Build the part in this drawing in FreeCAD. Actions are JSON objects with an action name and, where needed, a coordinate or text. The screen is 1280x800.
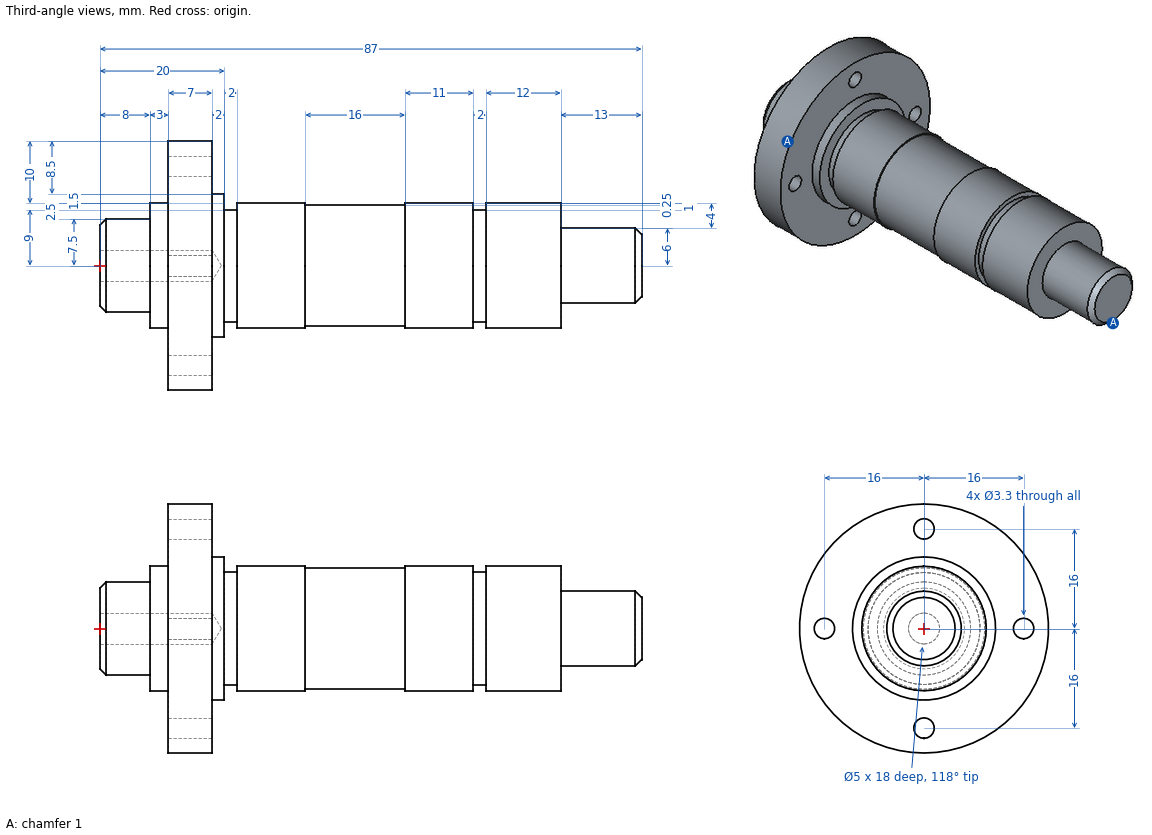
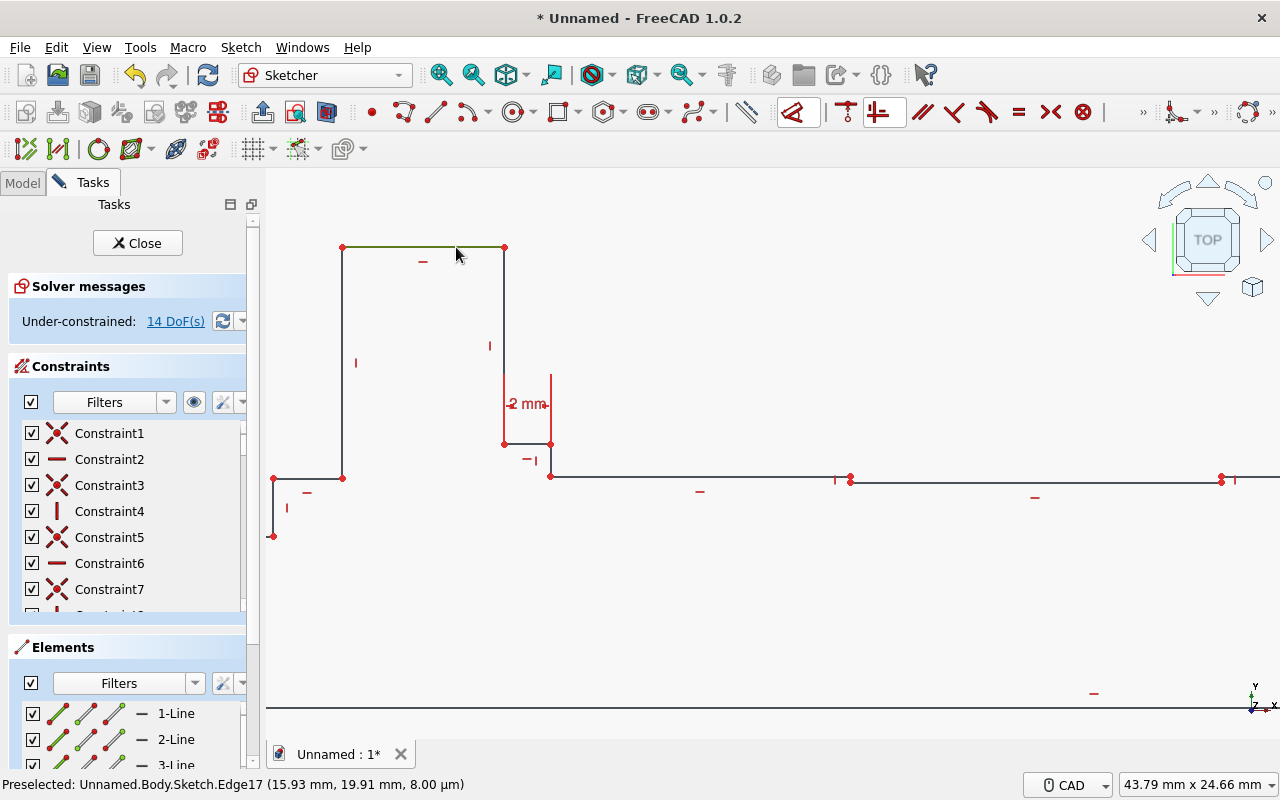
{"action": "left_click", "coordinate": [814, 112]}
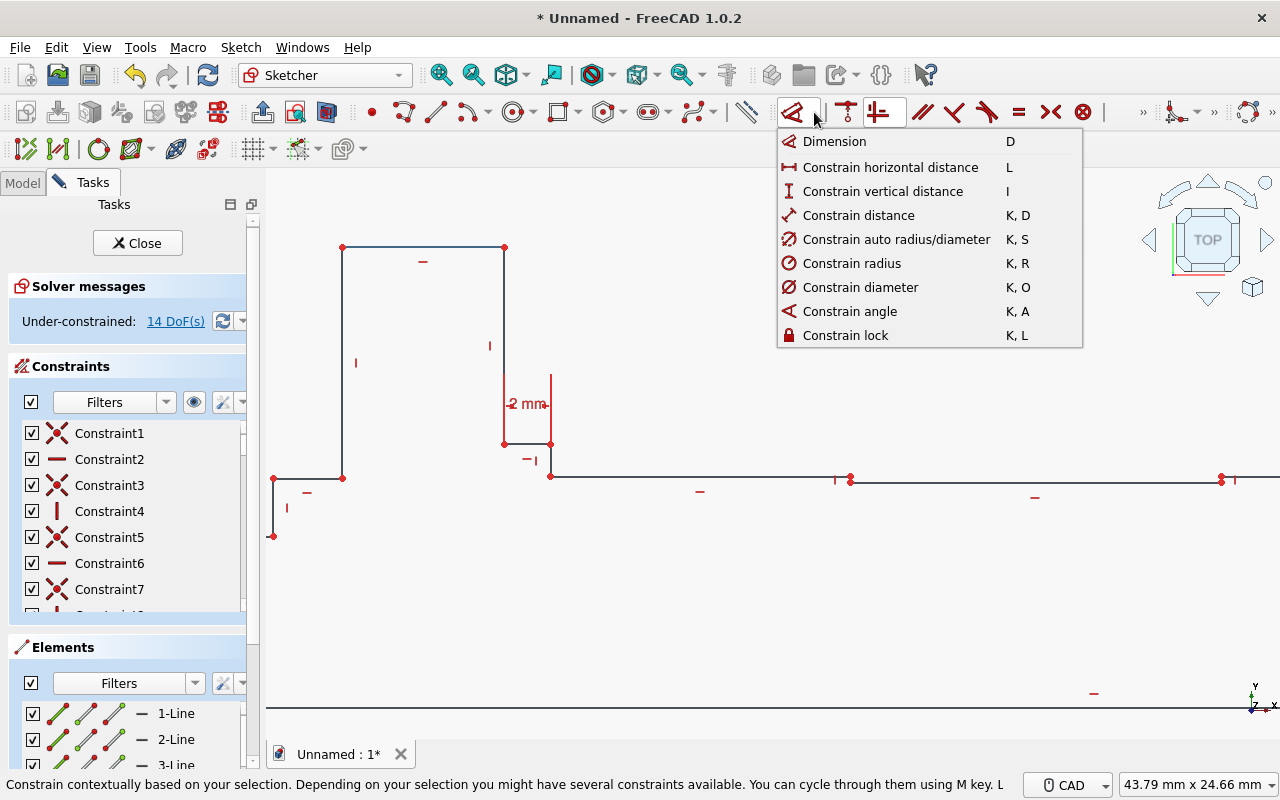
{"action": "left_click", "coordinate": [930, 167]}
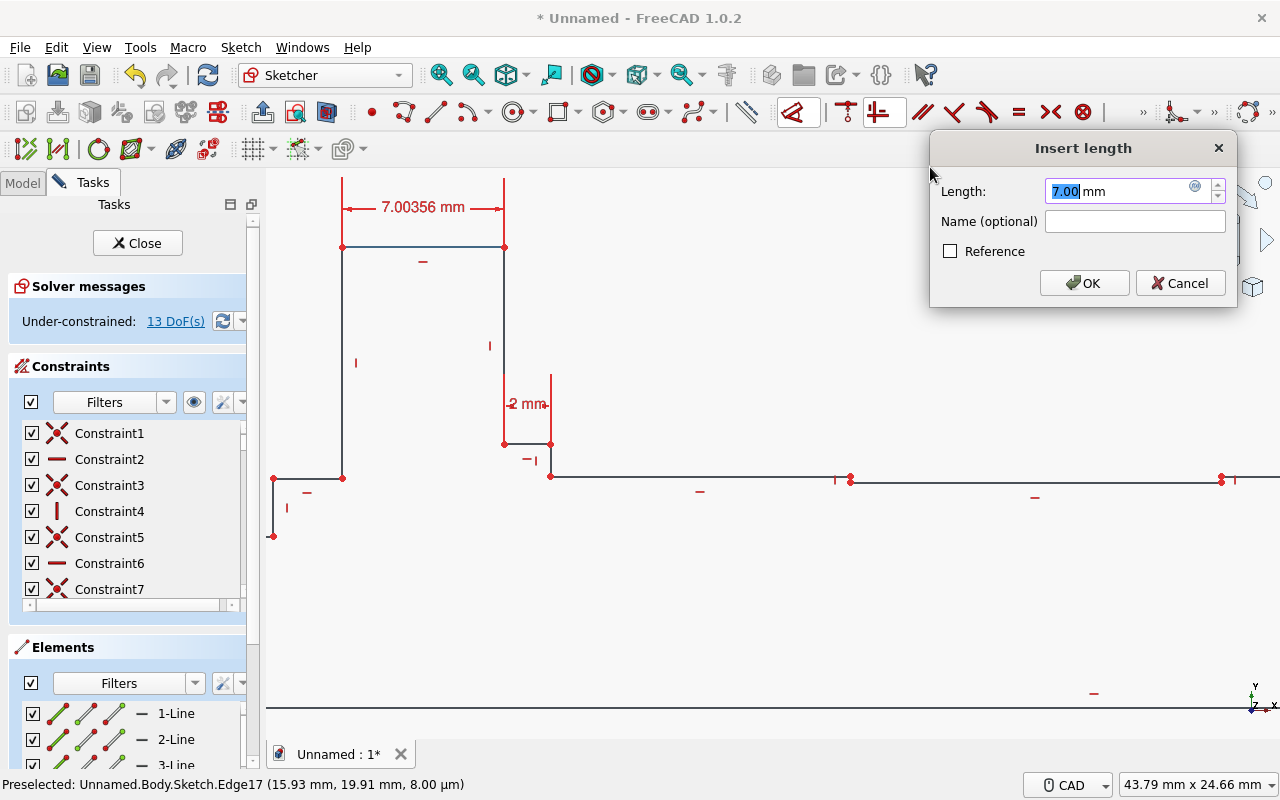
{"action": "type", "text": "7"}
{"action": "key", "text": "Return"}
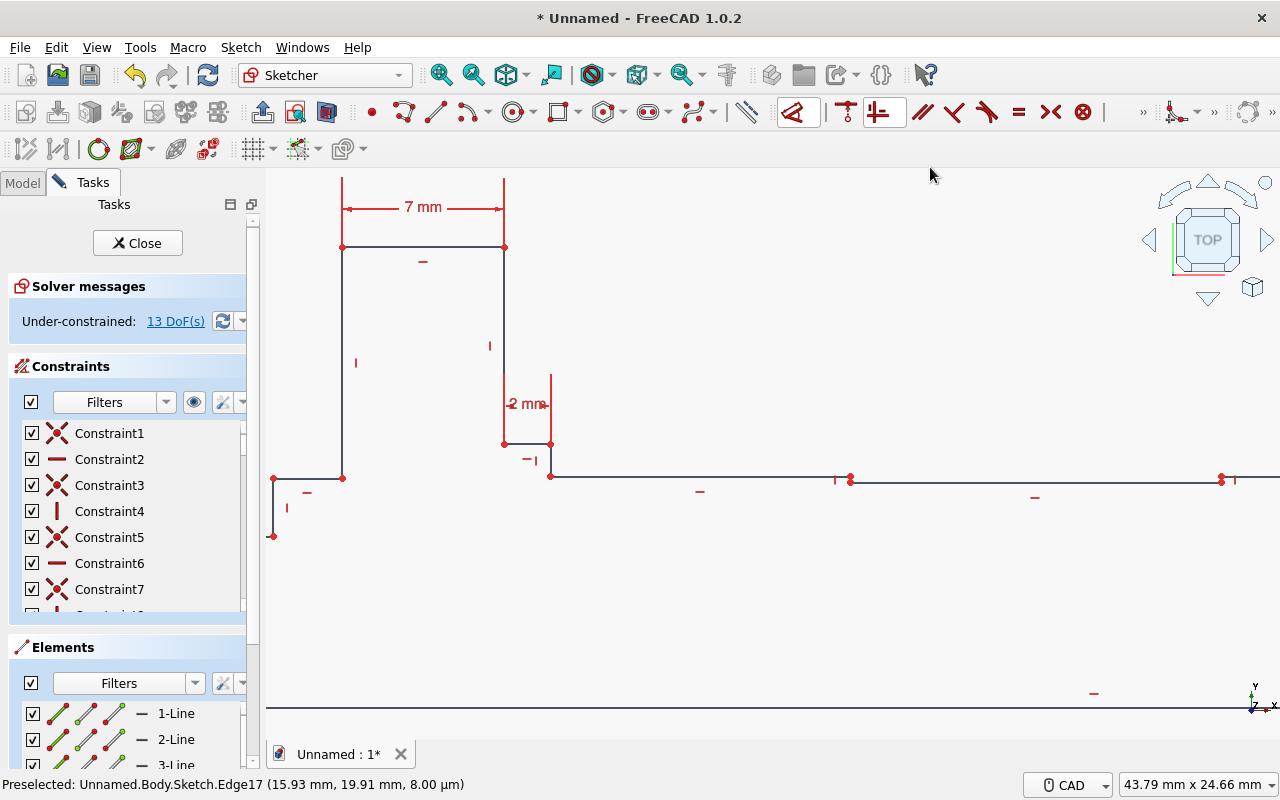
{"action": "left_click", "coordinate": [321, 479]}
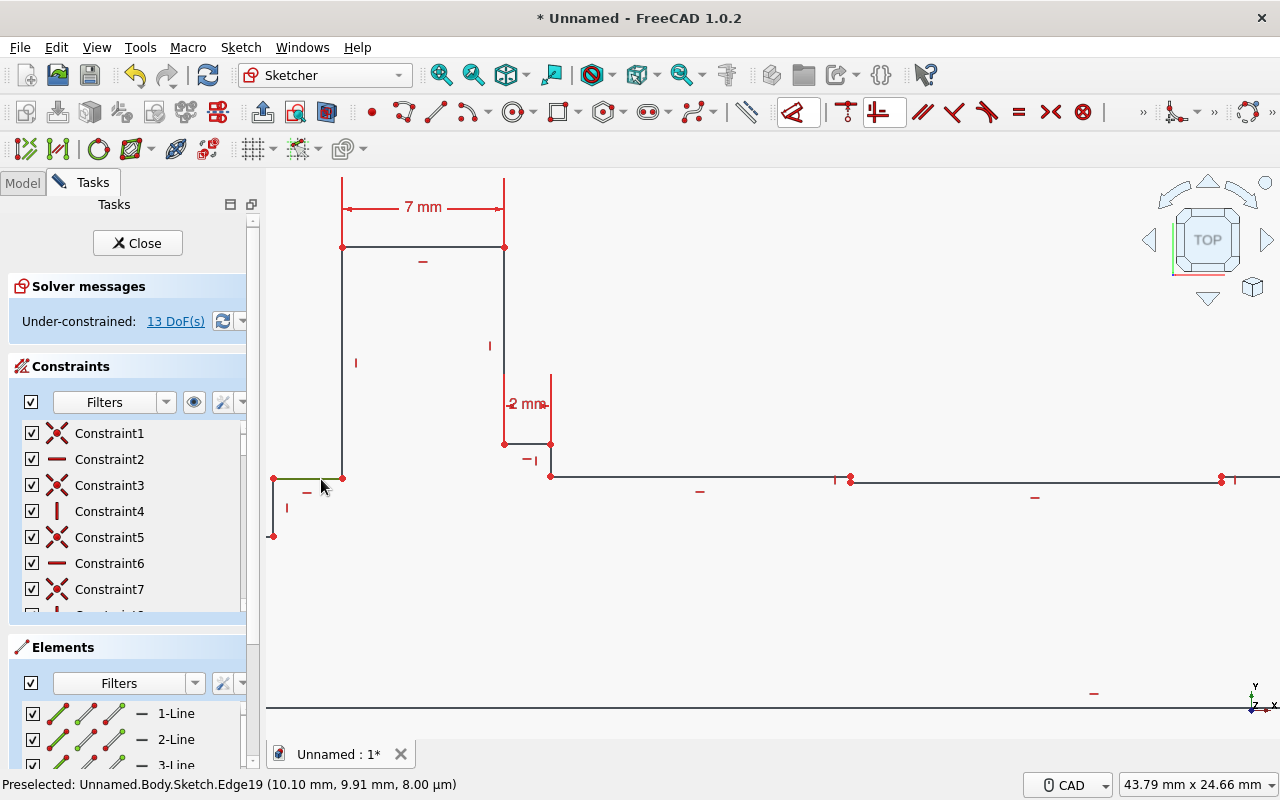
{"action": "key", "text": "l"}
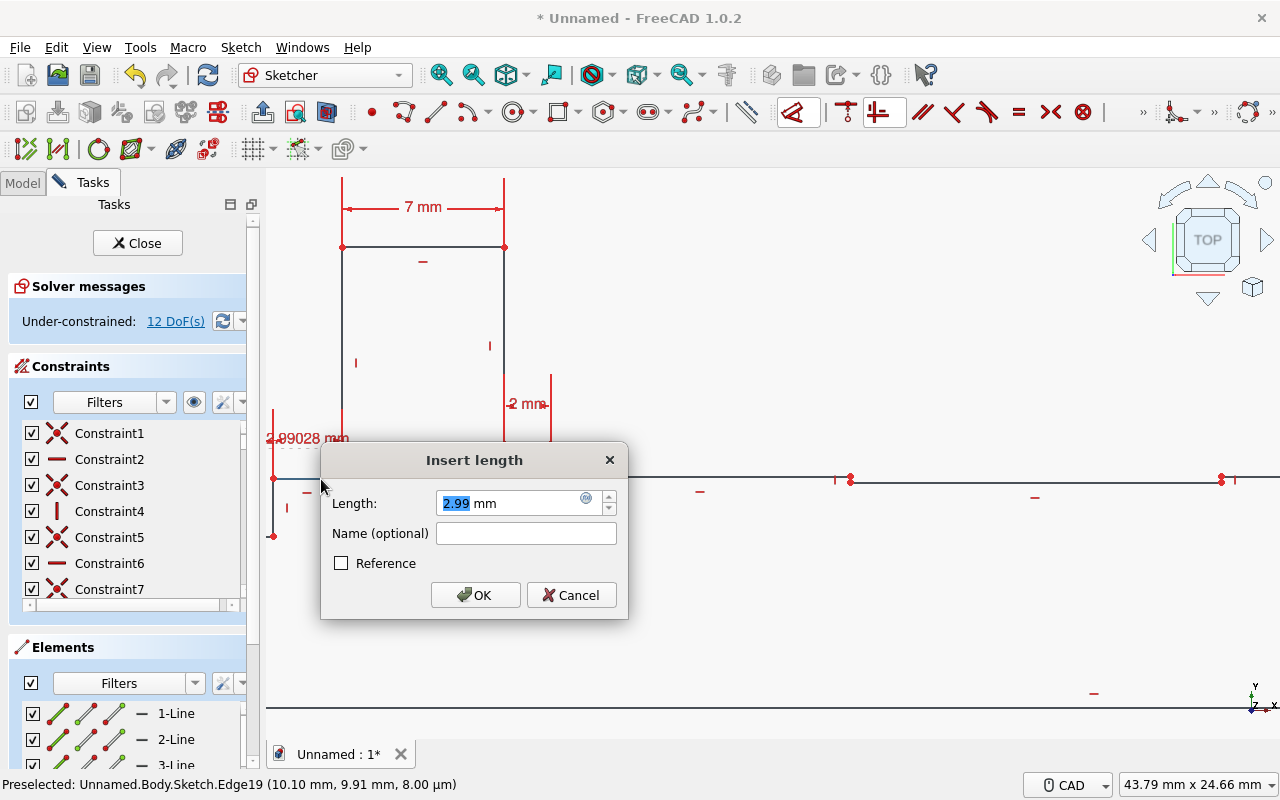
{"action": "type", "text": "3"}
{"action": "key", "text": "Return"}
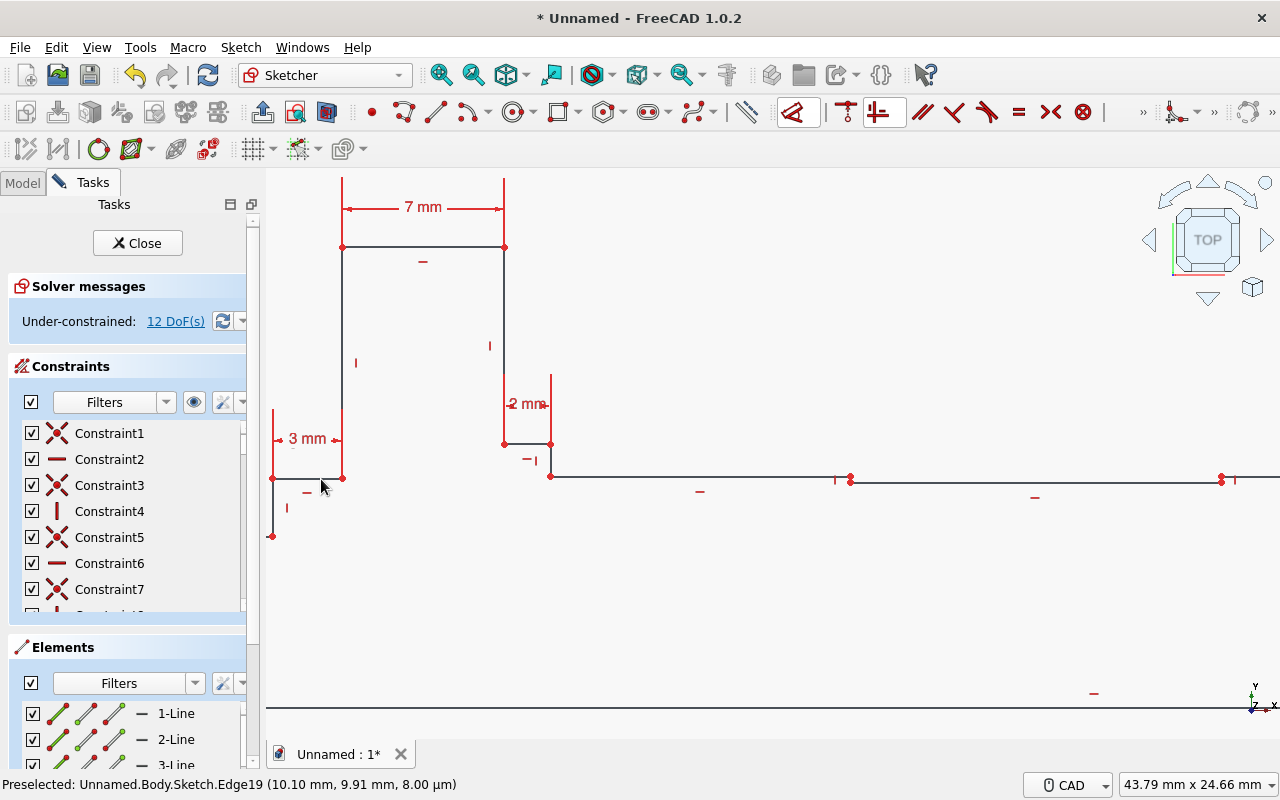
{"action": "scroll", "coordinate": [536, 444], "scroll_direction": "down", "scroll_amount": 6}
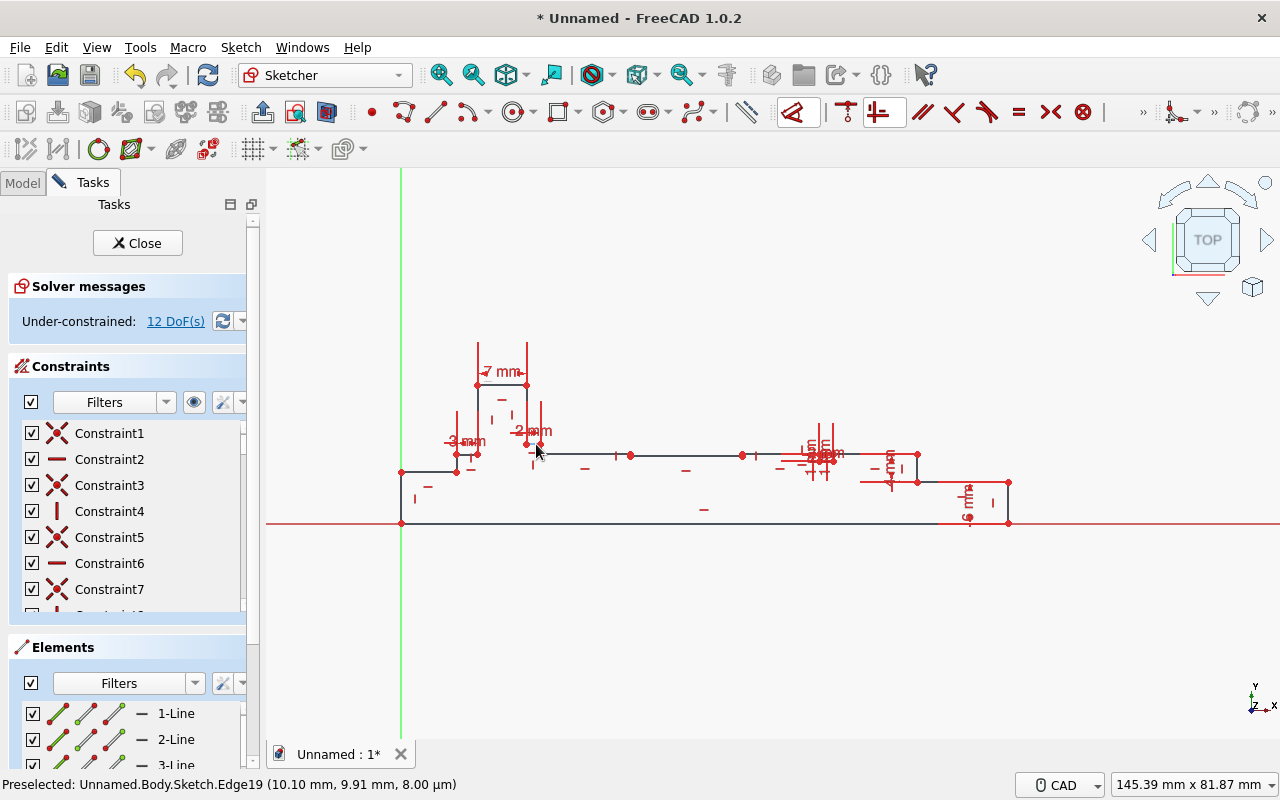
{"action": "left_click", "coordinate": [440, 472]}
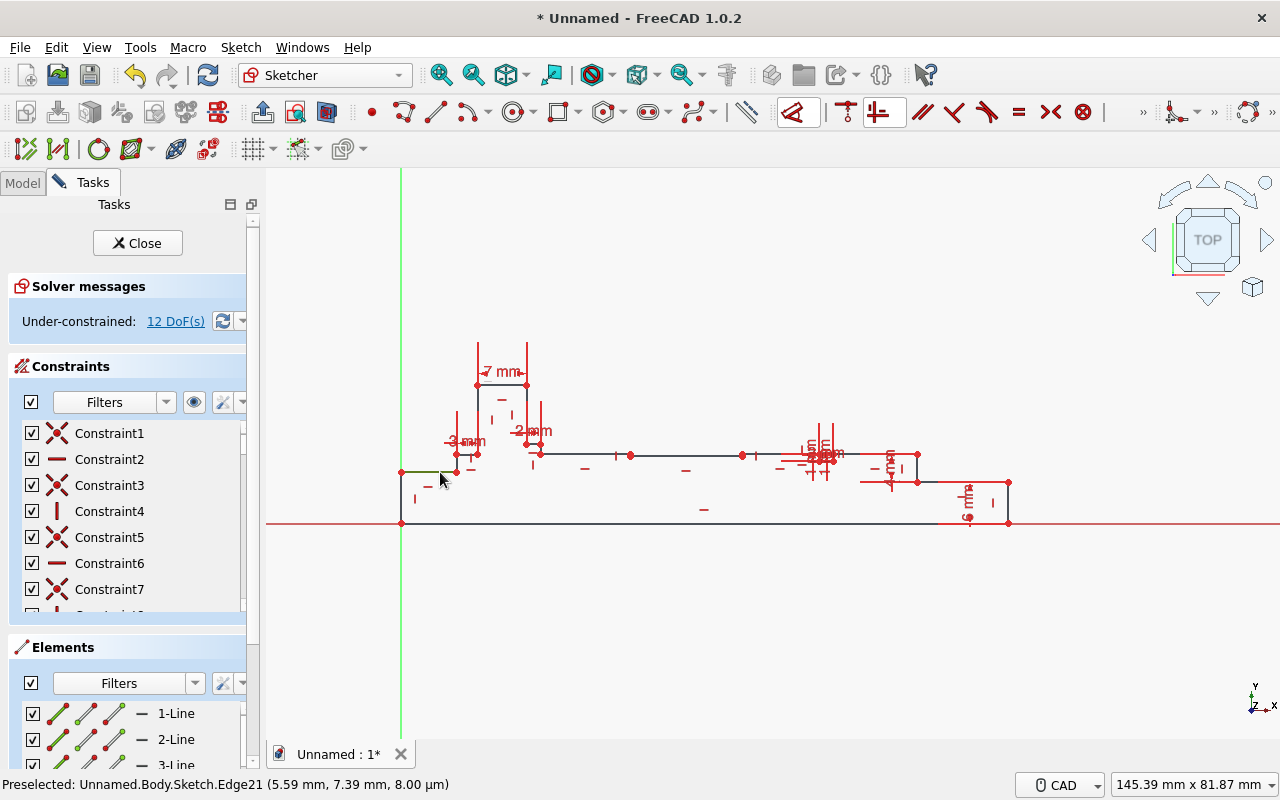
{"action": "key", "text": "l"}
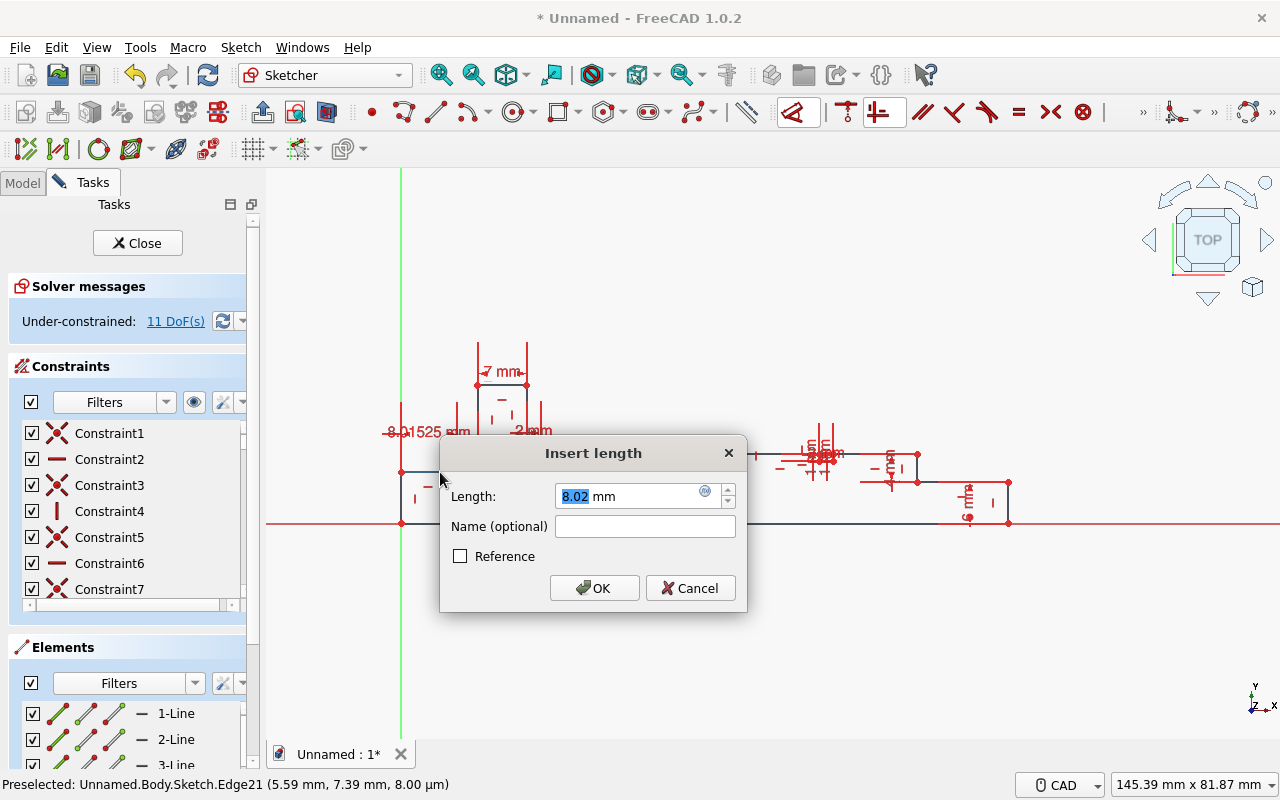
{"action": "type", "text": "8"}
{"action": "key", "text": "Return"}